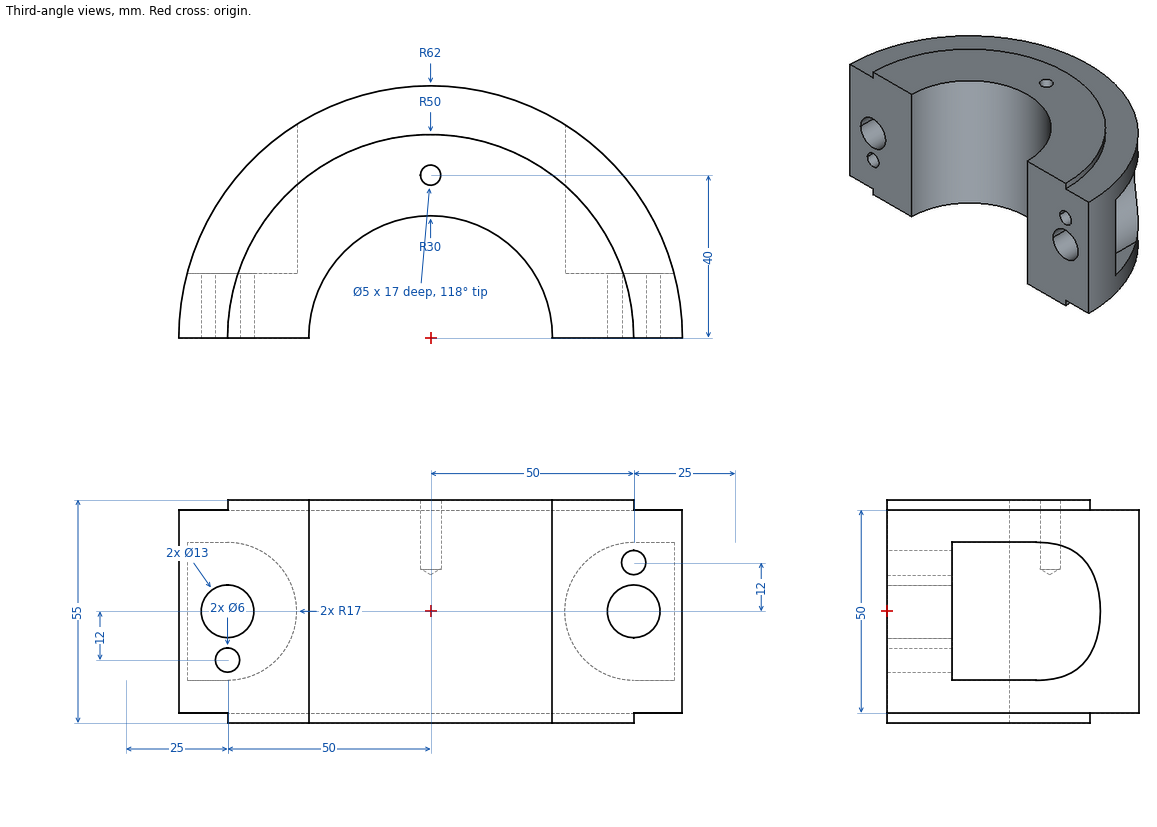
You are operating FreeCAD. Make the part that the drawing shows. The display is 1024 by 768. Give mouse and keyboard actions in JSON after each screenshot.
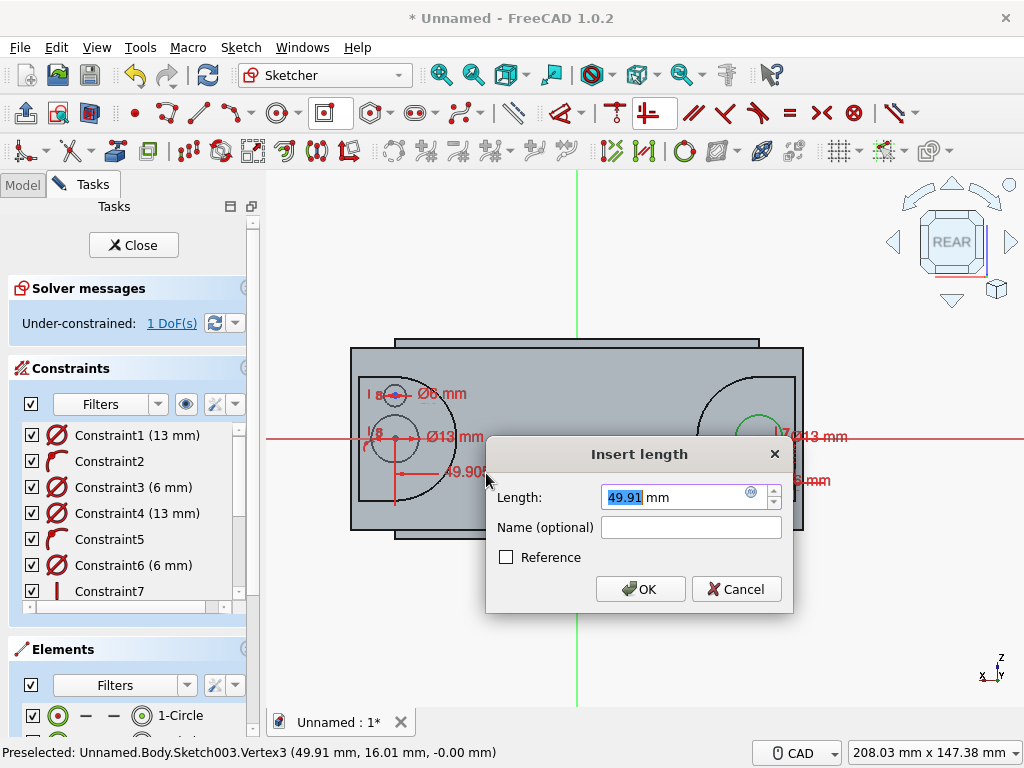
{"action": "type", "text": "50"}
{"action": "key", "text": "Return"}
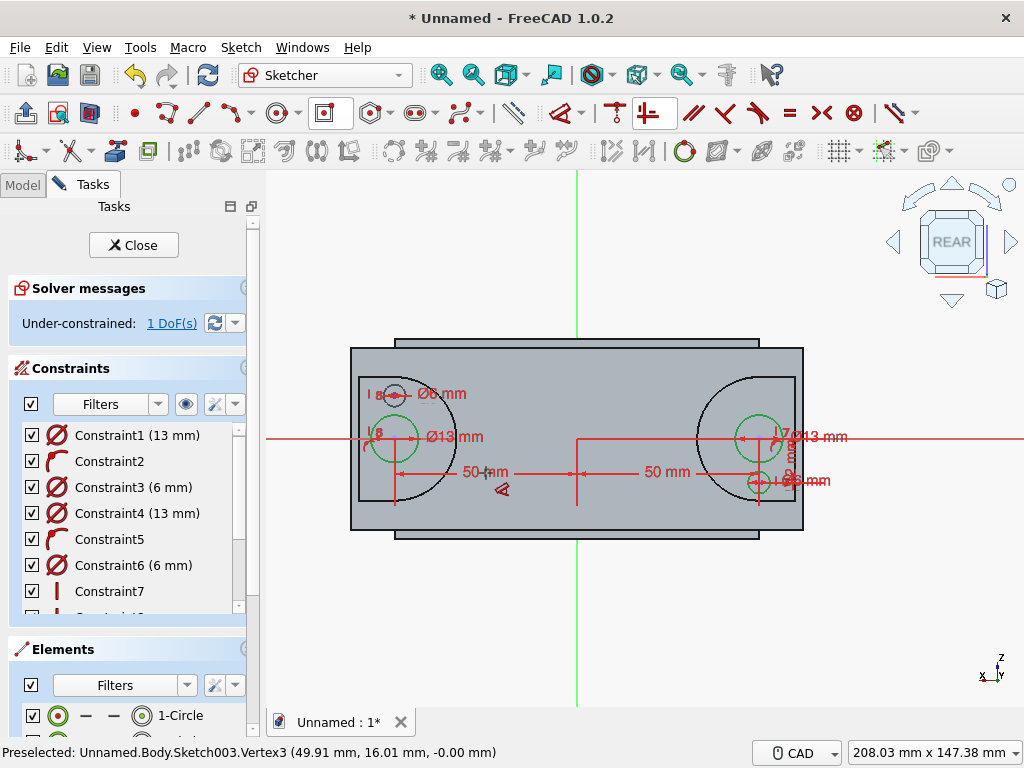
{"action": "left_click", "coordinate": [395, 396]}
{"action": "left_click", "coordinate": [361, 417]}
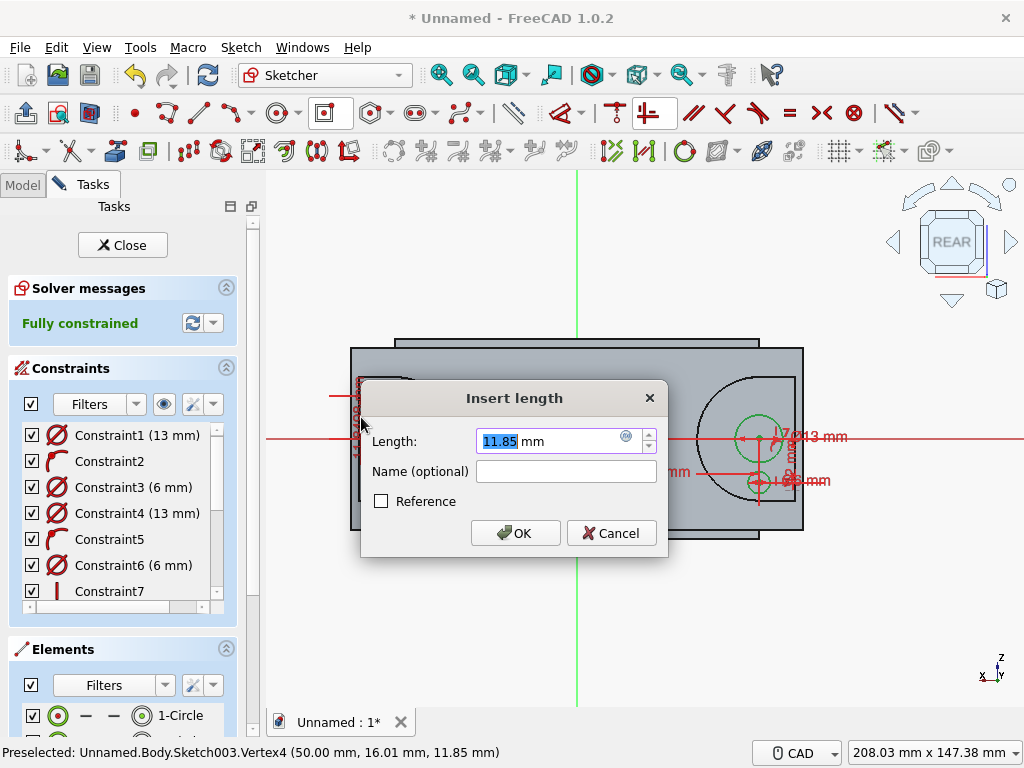
{"action": "type", "text": "12"}
{"action": "key", "text": "Return"}
{"action": "key", "text": "Escape"}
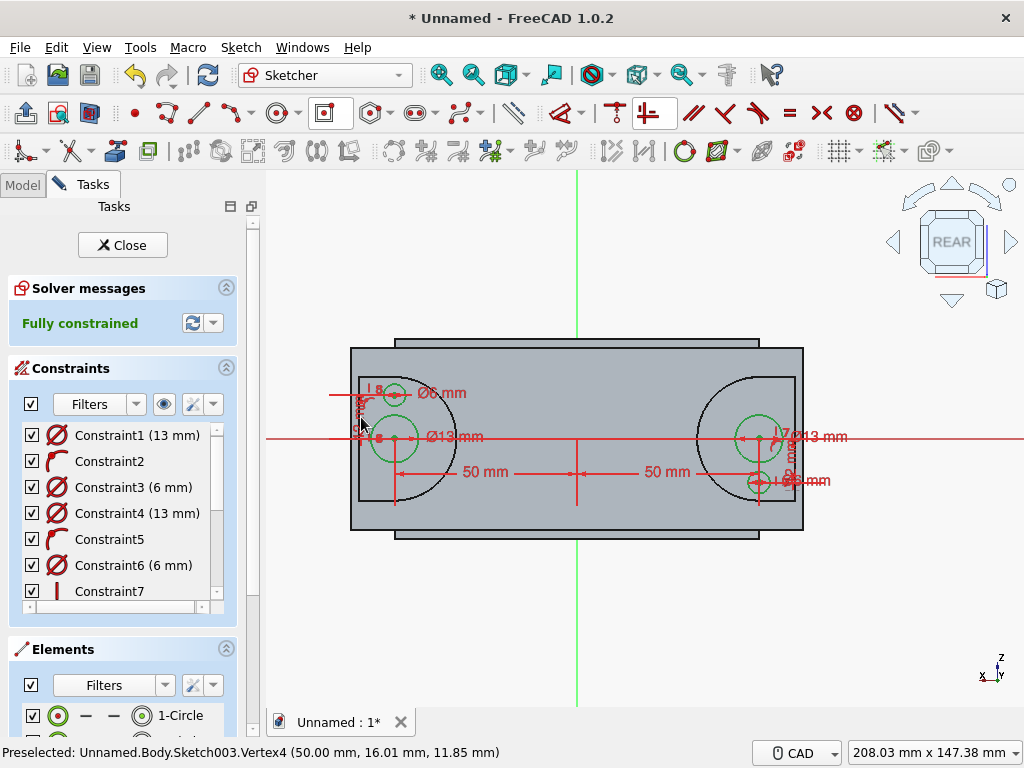
{"action": "left_click", "coordinate": [123, 245]}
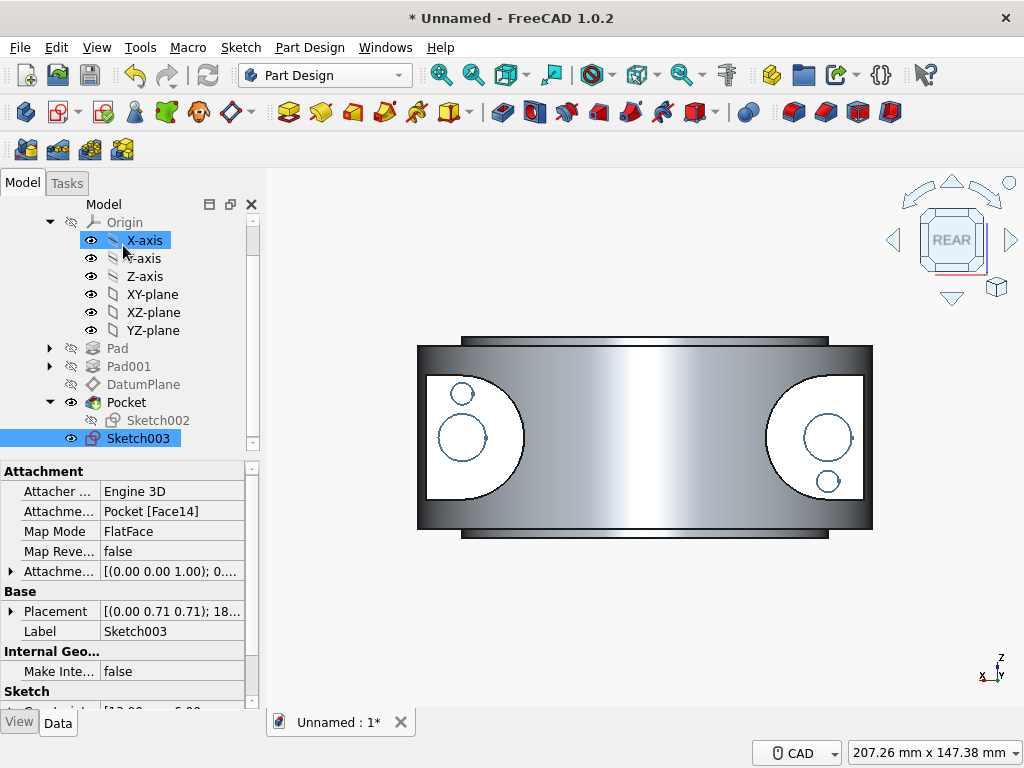
{"action": "left_click", "coordinate": [504, 112]}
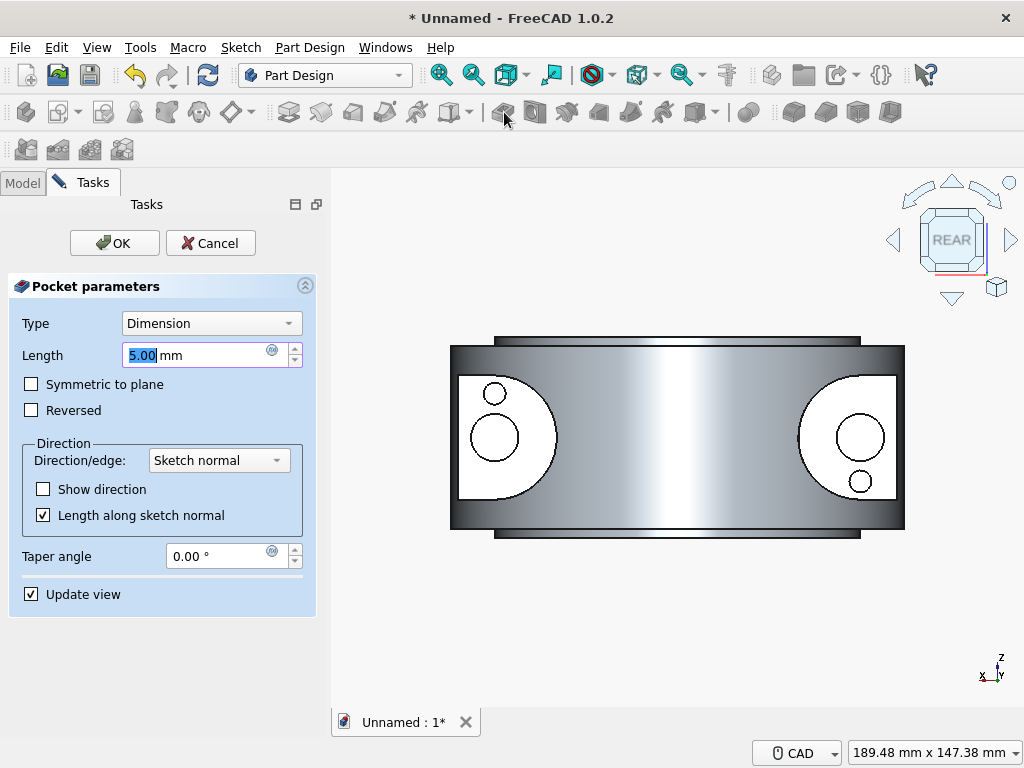
{"action": "left_click", "coordinate": [212, 324]}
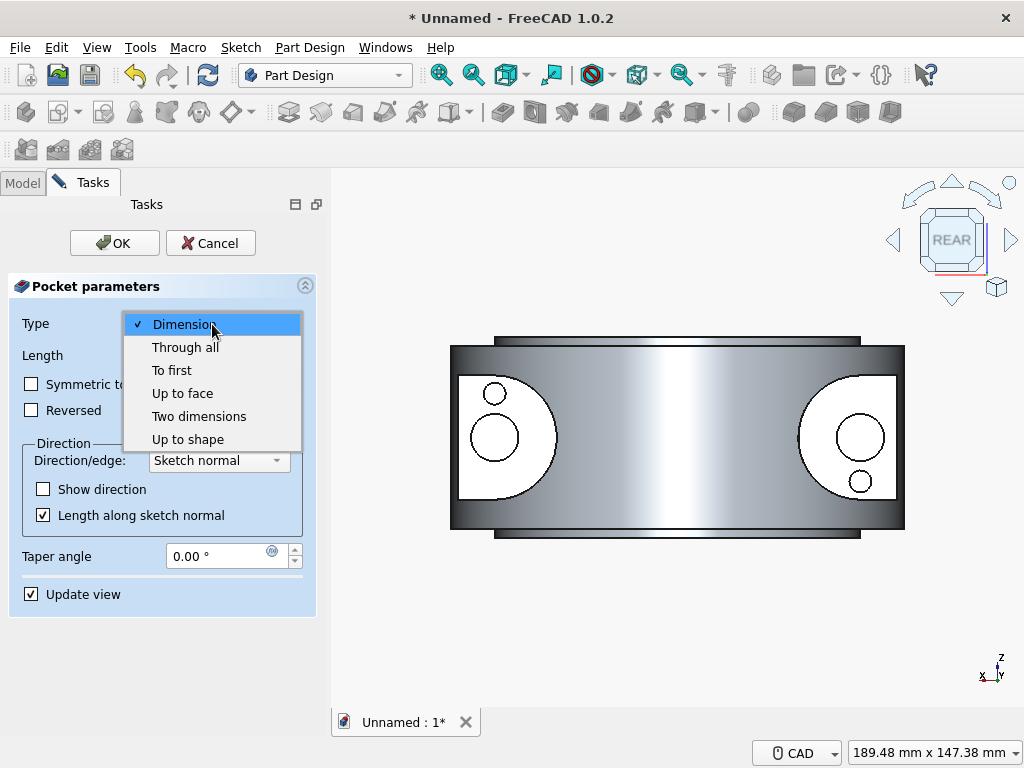
{"action": "left_click", "coordinate": [212, 348]}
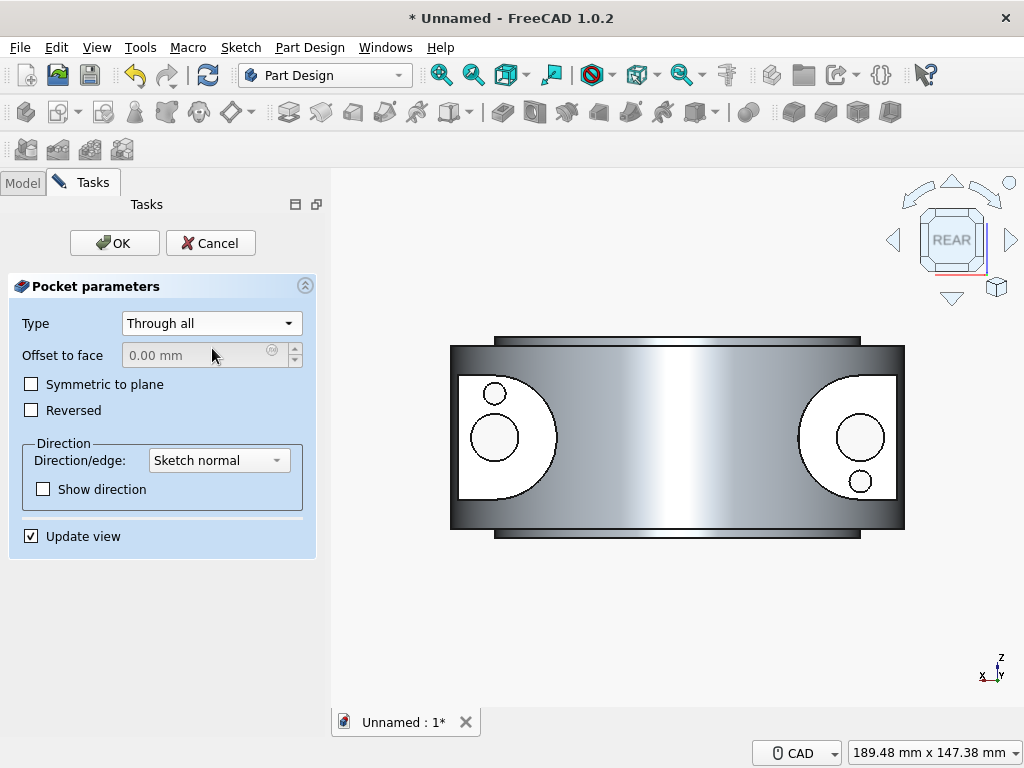
{"action": "left_click", "coordinate": [115, 243]}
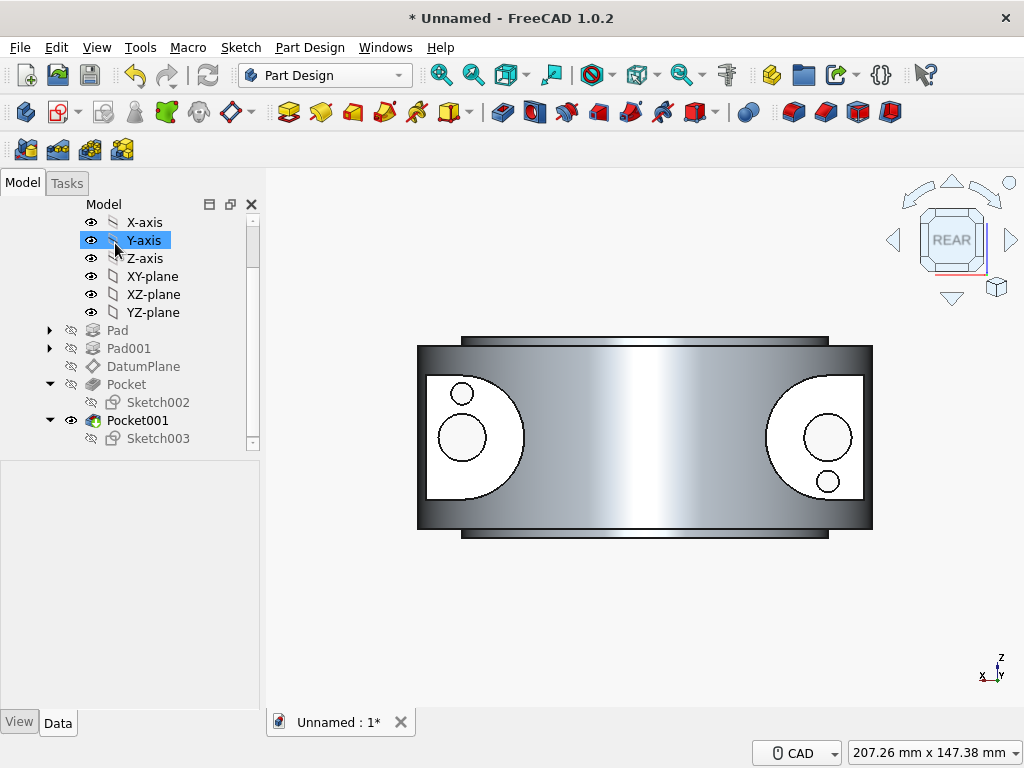
{"action": "key", "text": "0"}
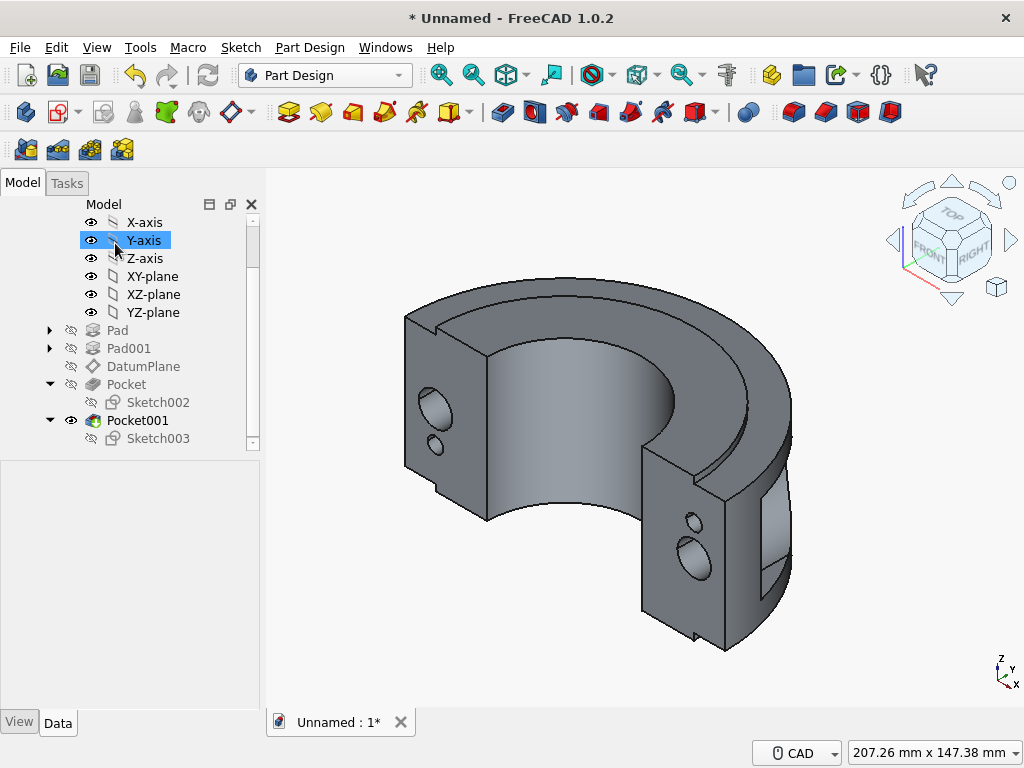
{"action": "left_click", "coordinate": [666, 342]}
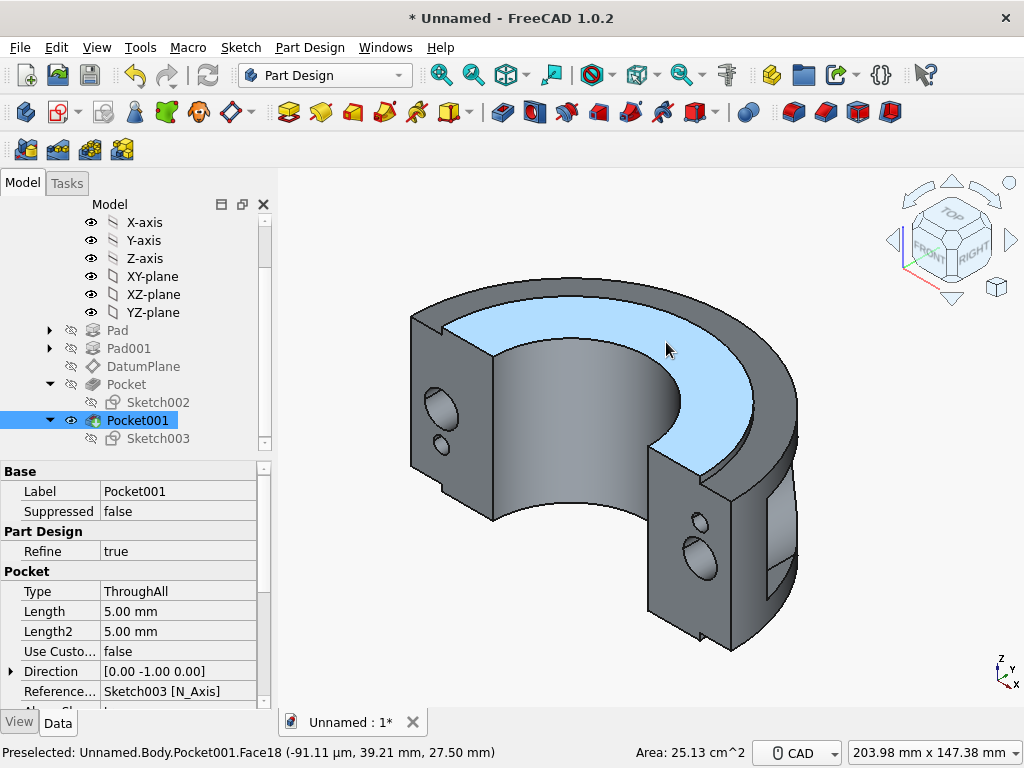
{"action": "left_click", "coordinate": [58, 112]}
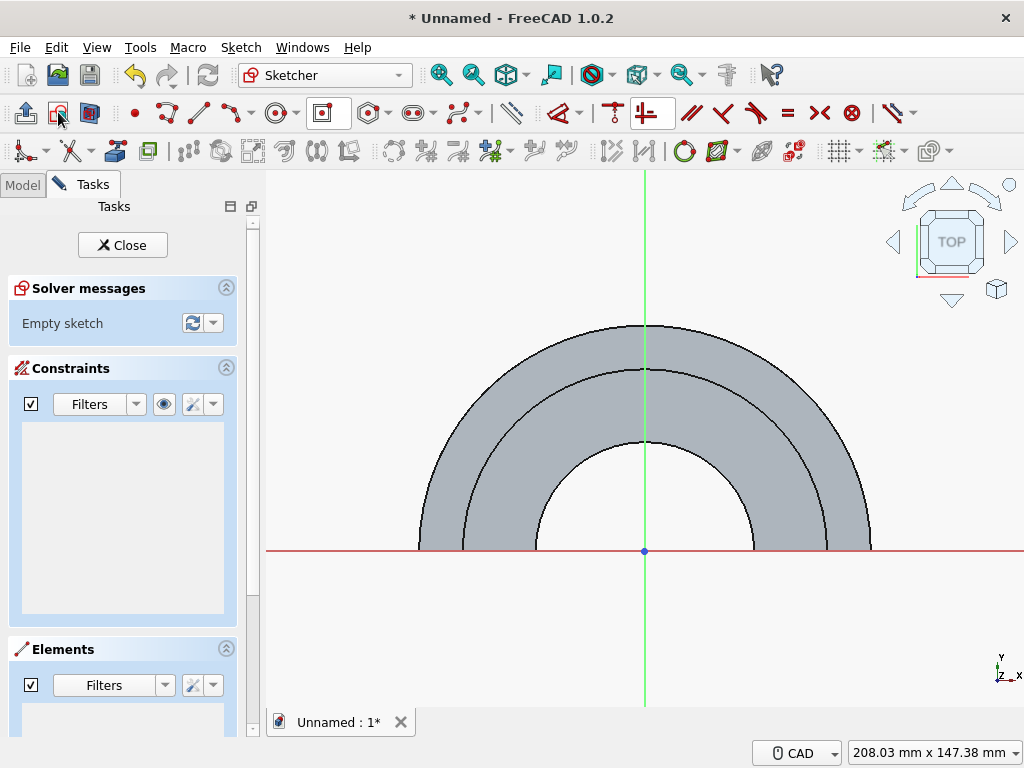
{"action": "scroll", "coordinate": [649, 404], "scroll_direction": "up", "scroll_amount": 15}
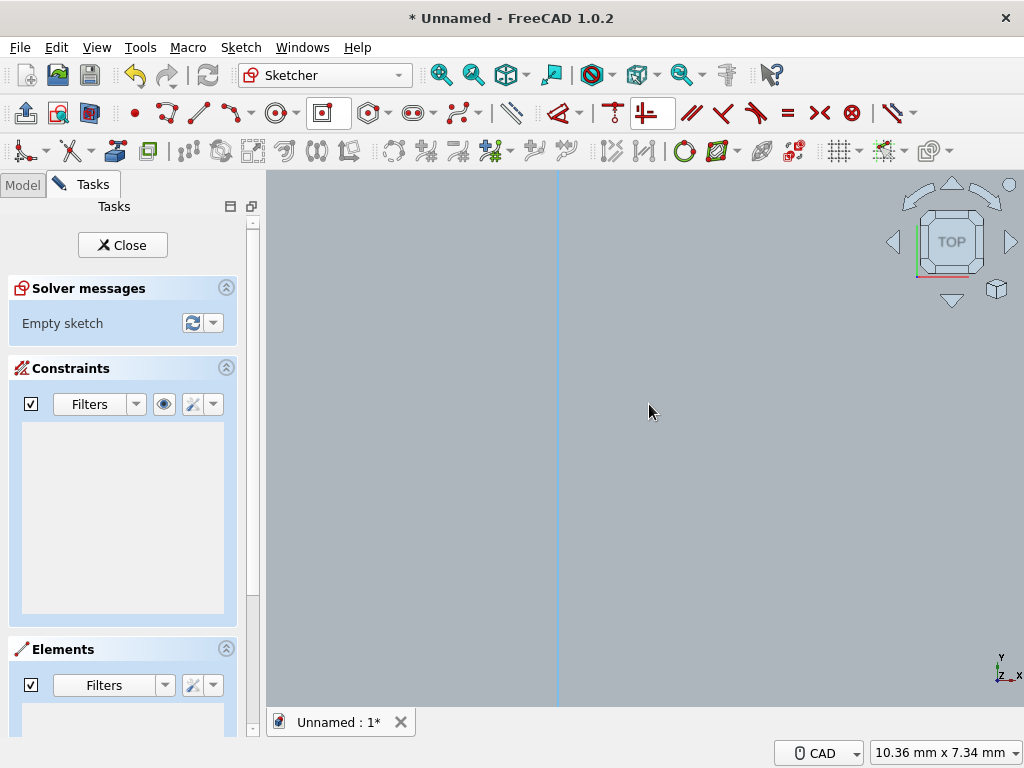
{"action": "left_click", "coordinate": [276, 114]}